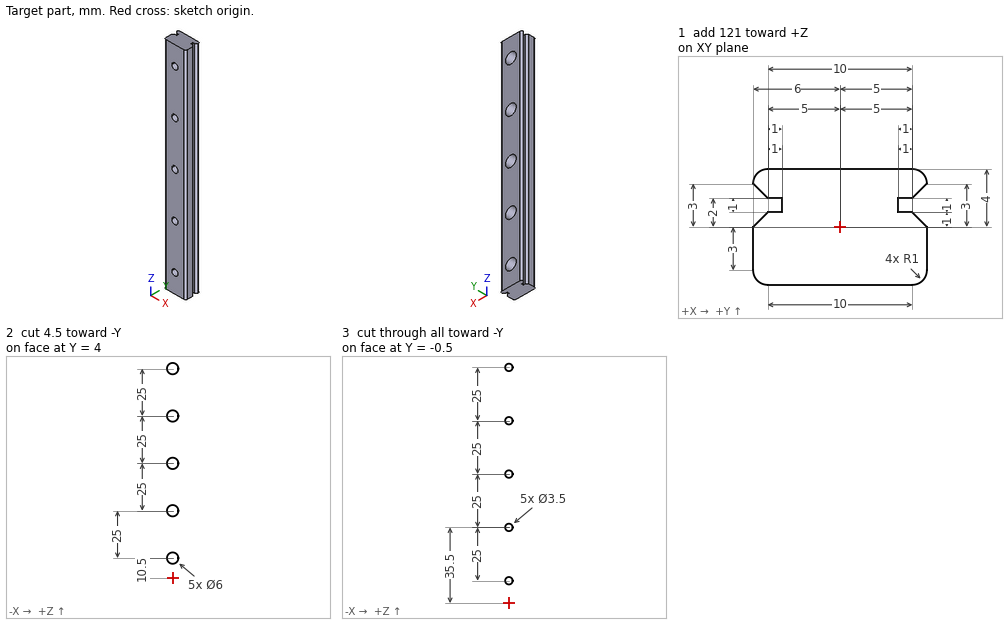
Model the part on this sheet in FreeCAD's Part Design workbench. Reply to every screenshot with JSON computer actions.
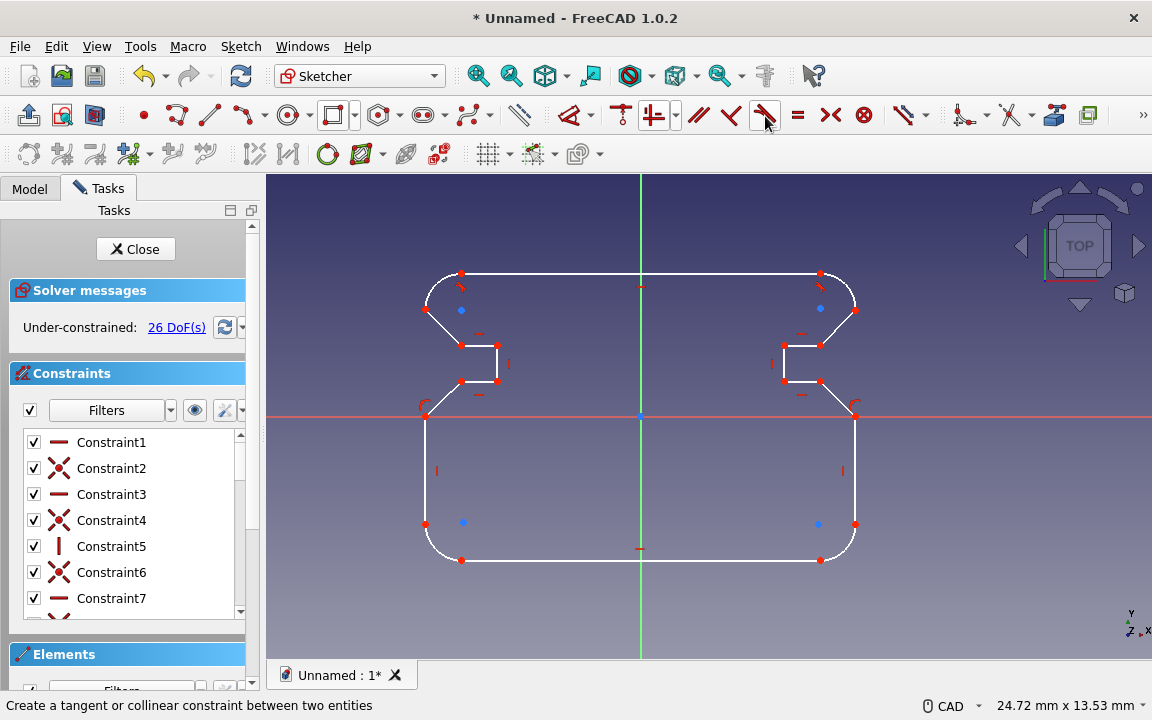
{"action": "left_click", "coordinate": [425, 449]}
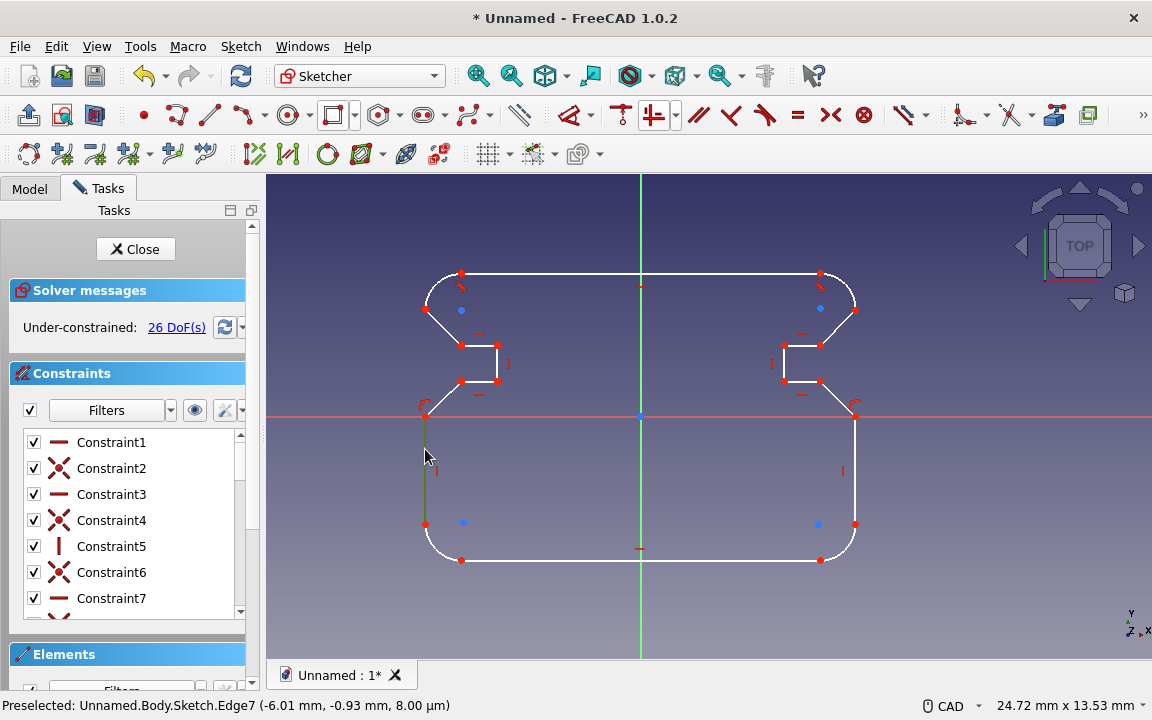
{"action": "left_click", "coordinate": [430, 541]}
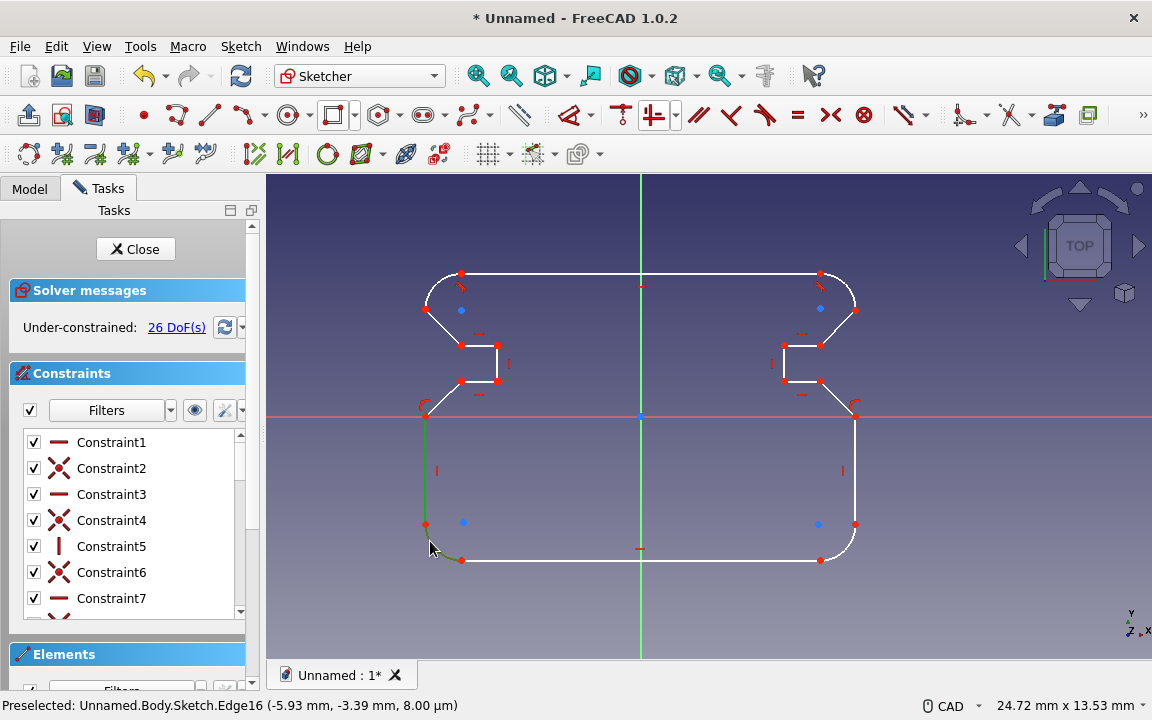
{"action": "left_click", "coordinate": [765, 116]}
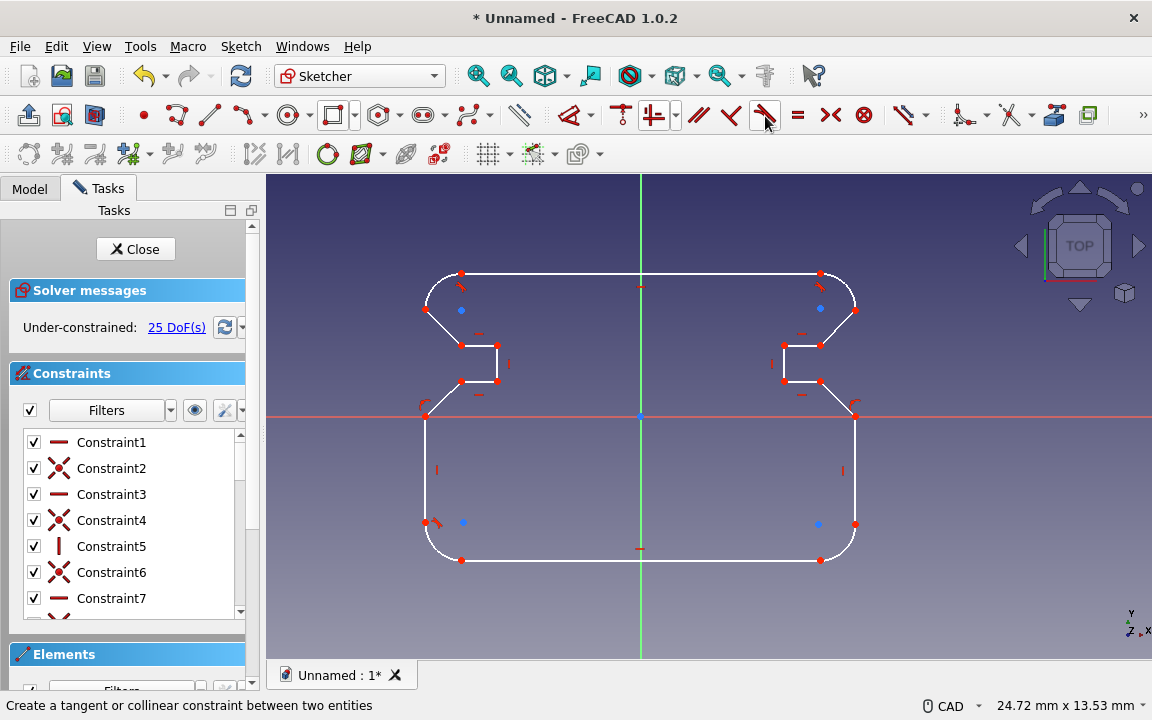
{"action": "left_click", "coordinate": [569, 561]}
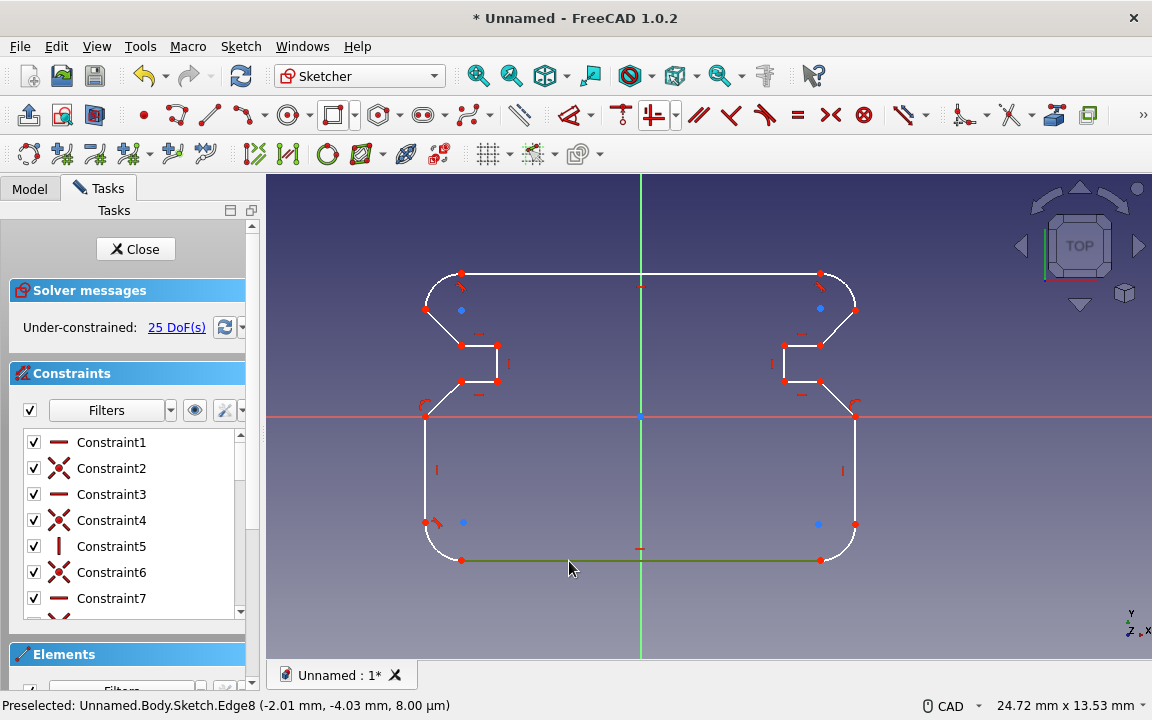
{"action": "left_click", "coordinate": [429, 540]}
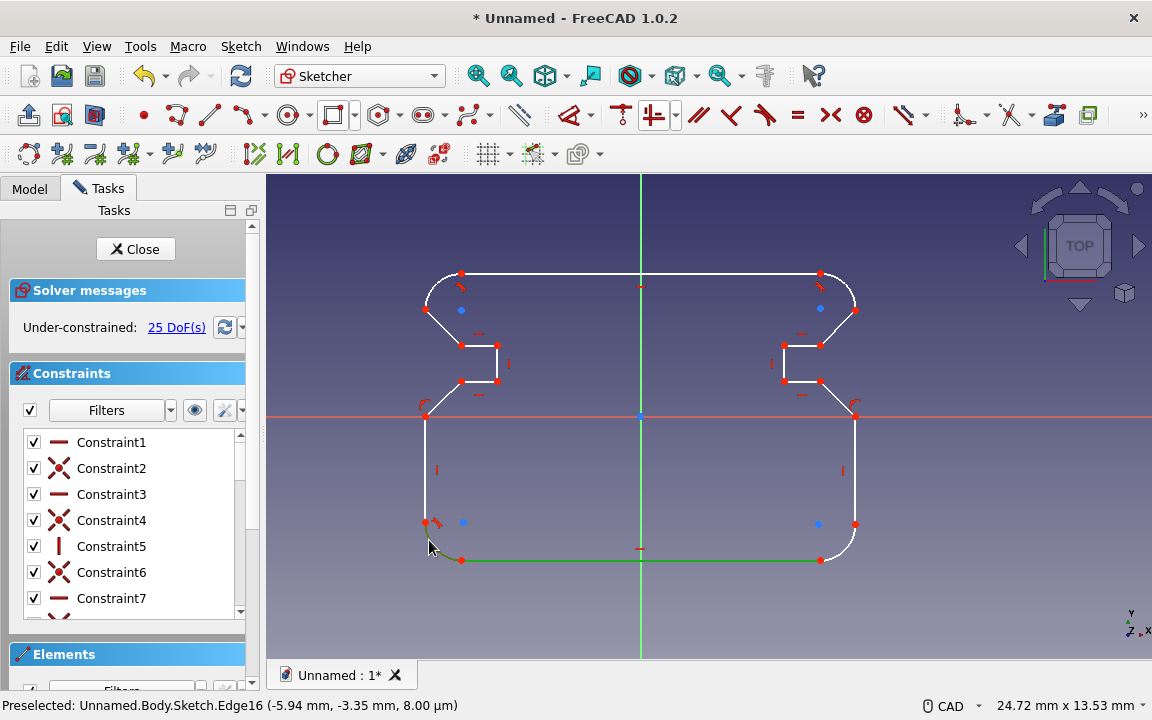
{"action": "left_click", "coordinate": [765, 116]}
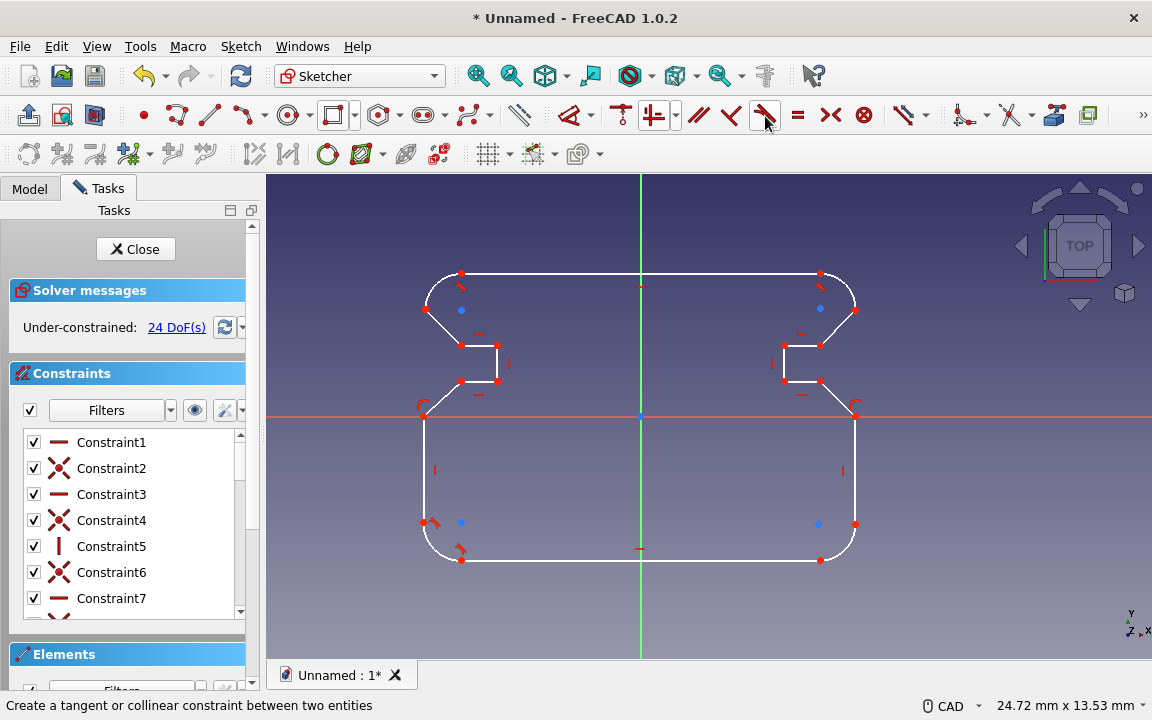
{"action": "left_click", "coordinate": [569, 561]}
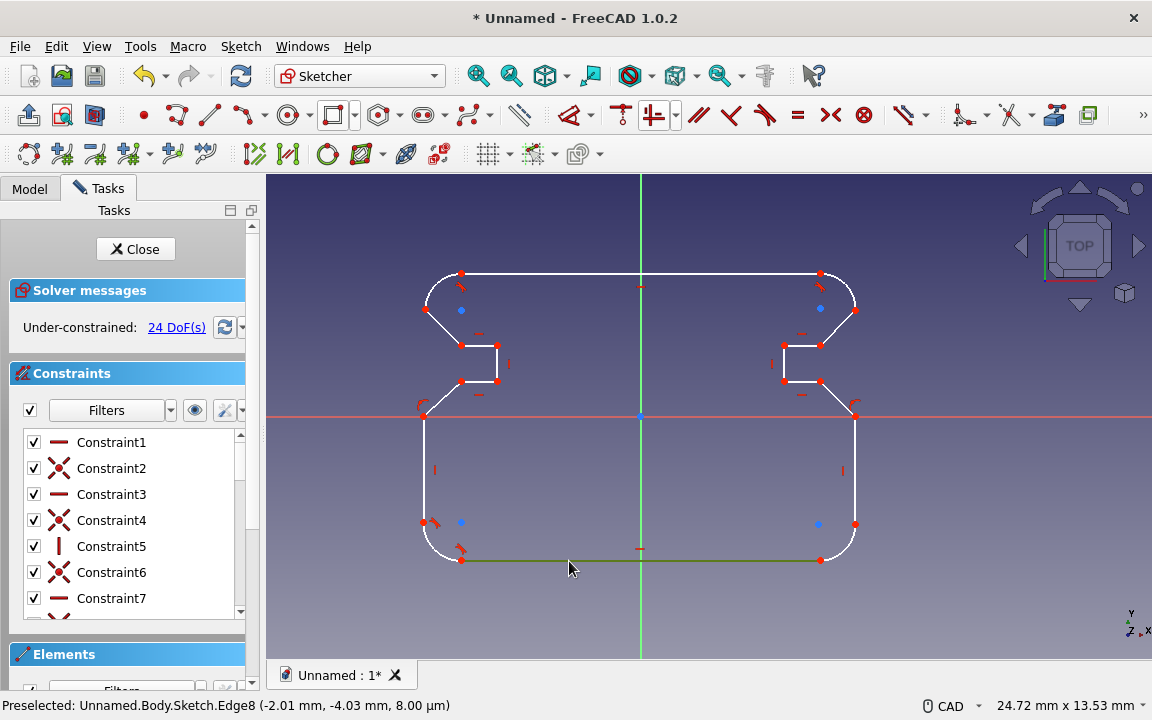
{"action": "left_click", "coordinate": [836, 556]}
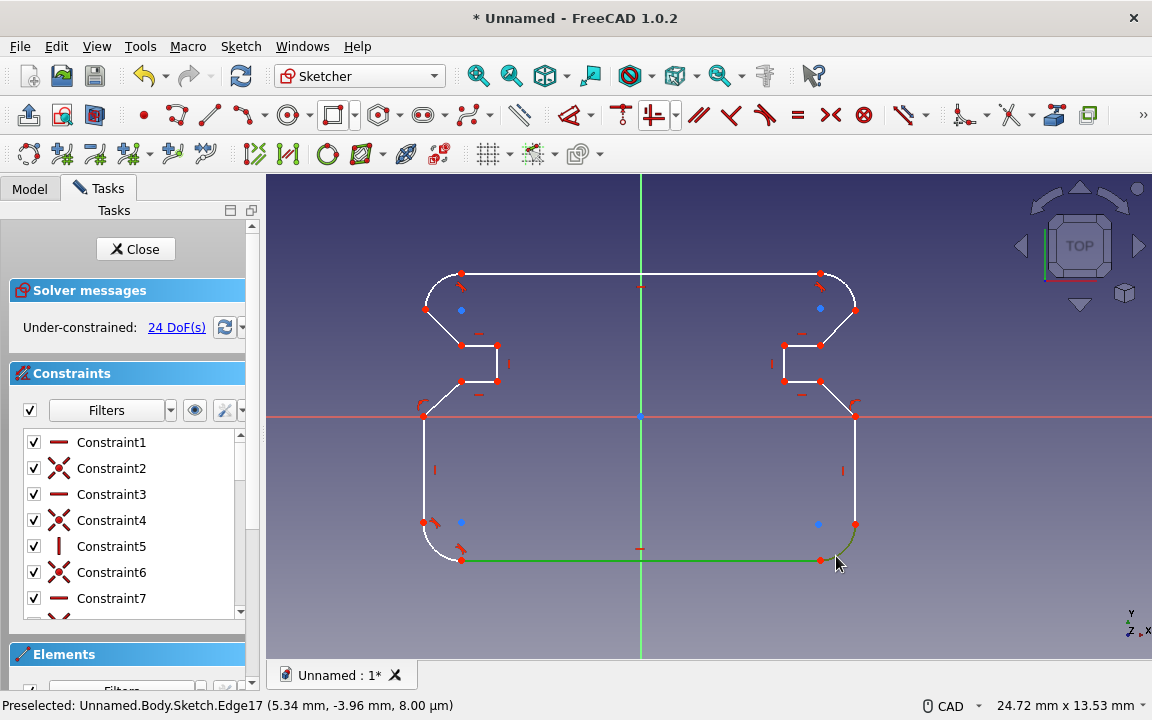
{"action": "left_click", "coordinate": [765, 116]}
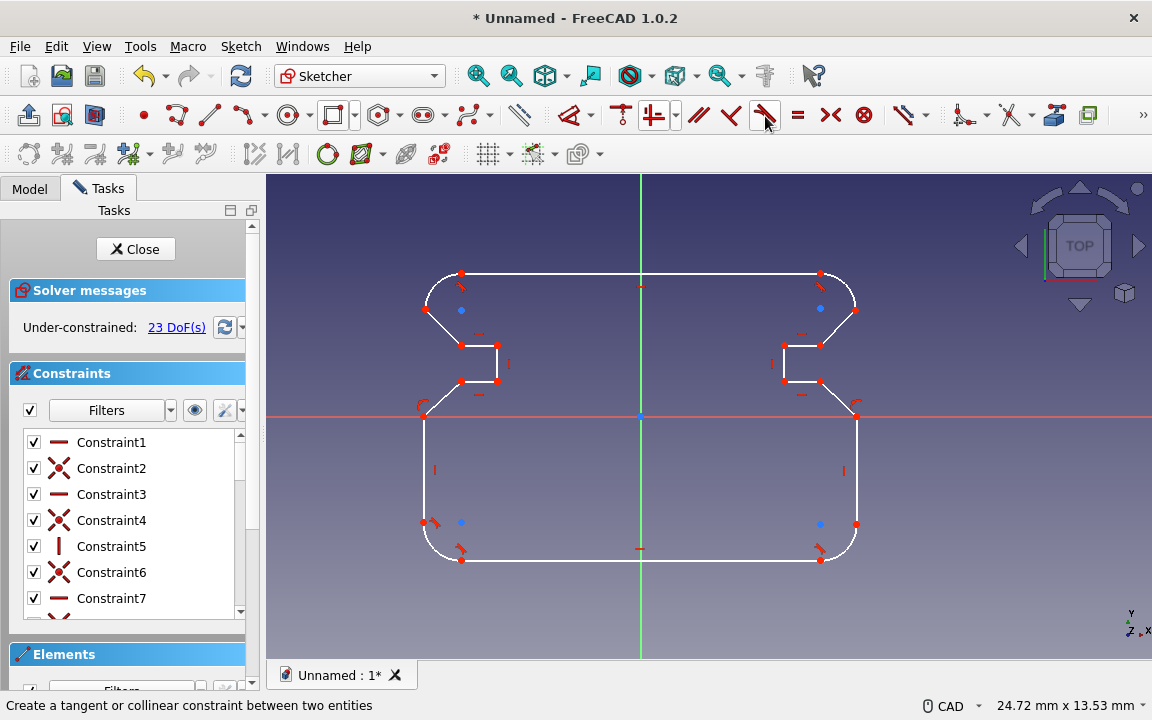
{"action": "left_click", "coordinate": [857, 492]}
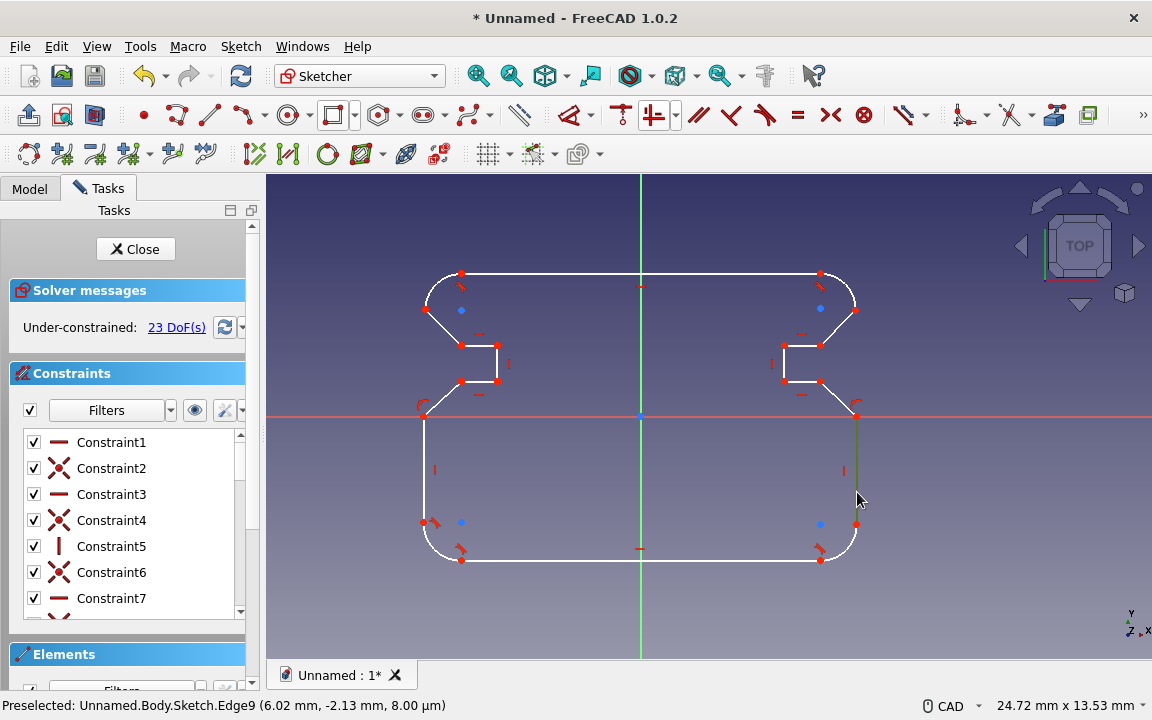
{"action": "left_click", "coordinate": [837, 557]}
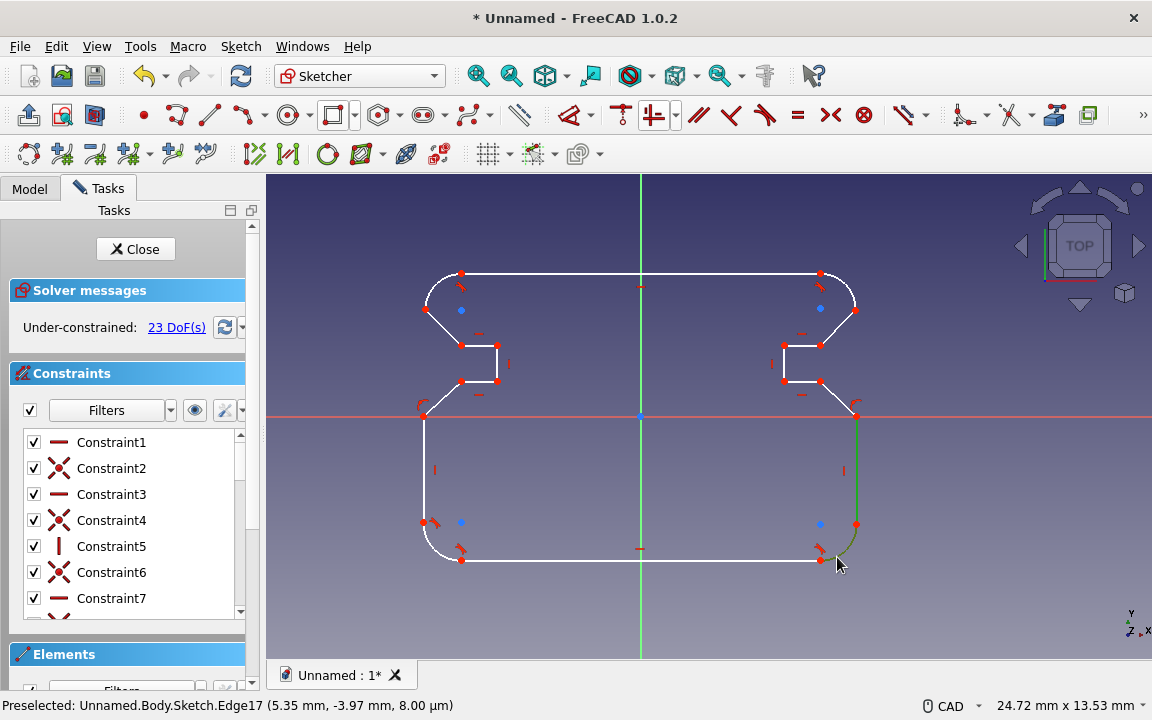
{"action": "left_click", "coordinate": [765, 116]}